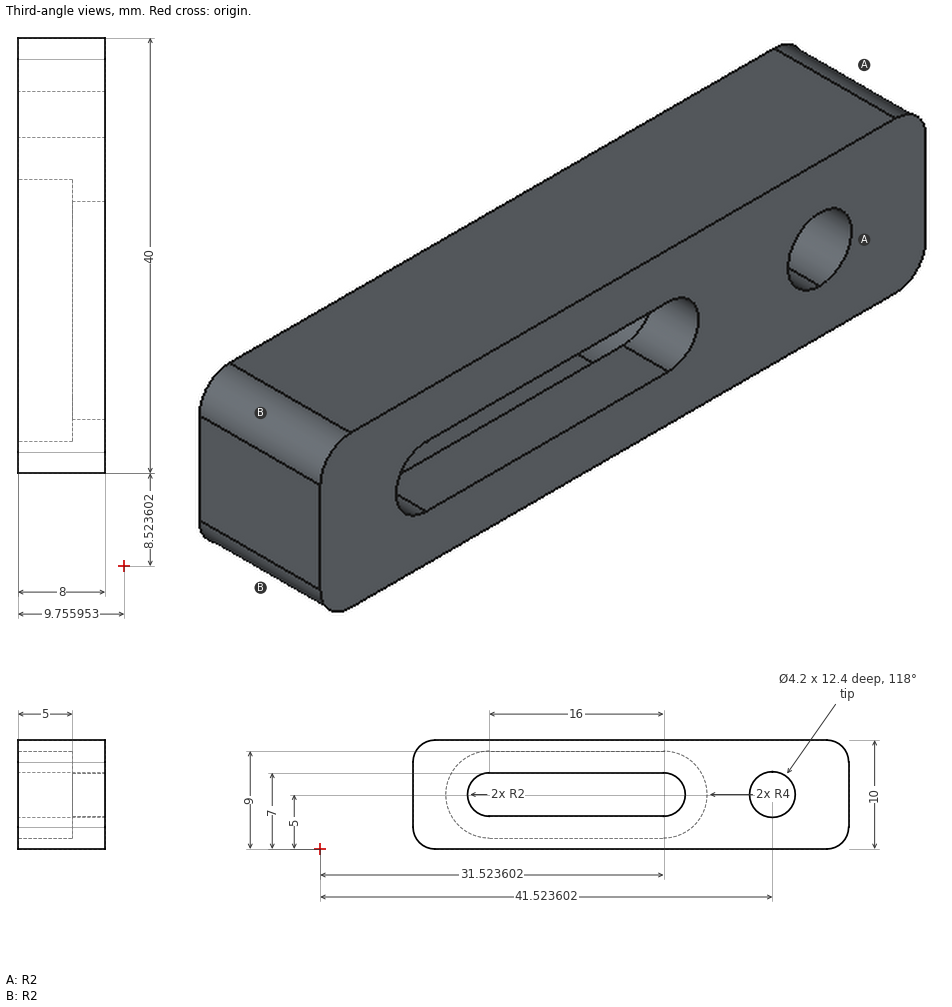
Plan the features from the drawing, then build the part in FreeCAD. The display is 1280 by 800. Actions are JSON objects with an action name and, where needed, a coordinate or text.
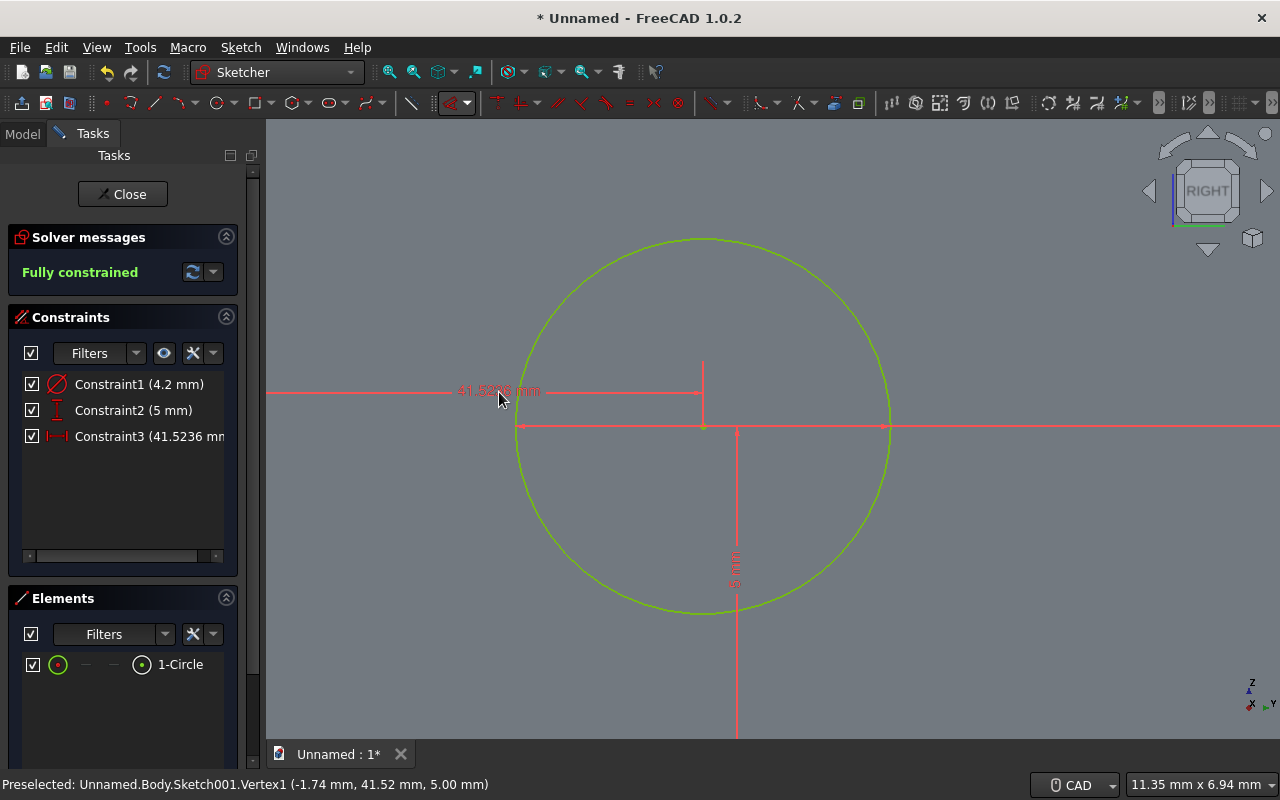
{"action": "left_click", "coordinate": [123, 194]}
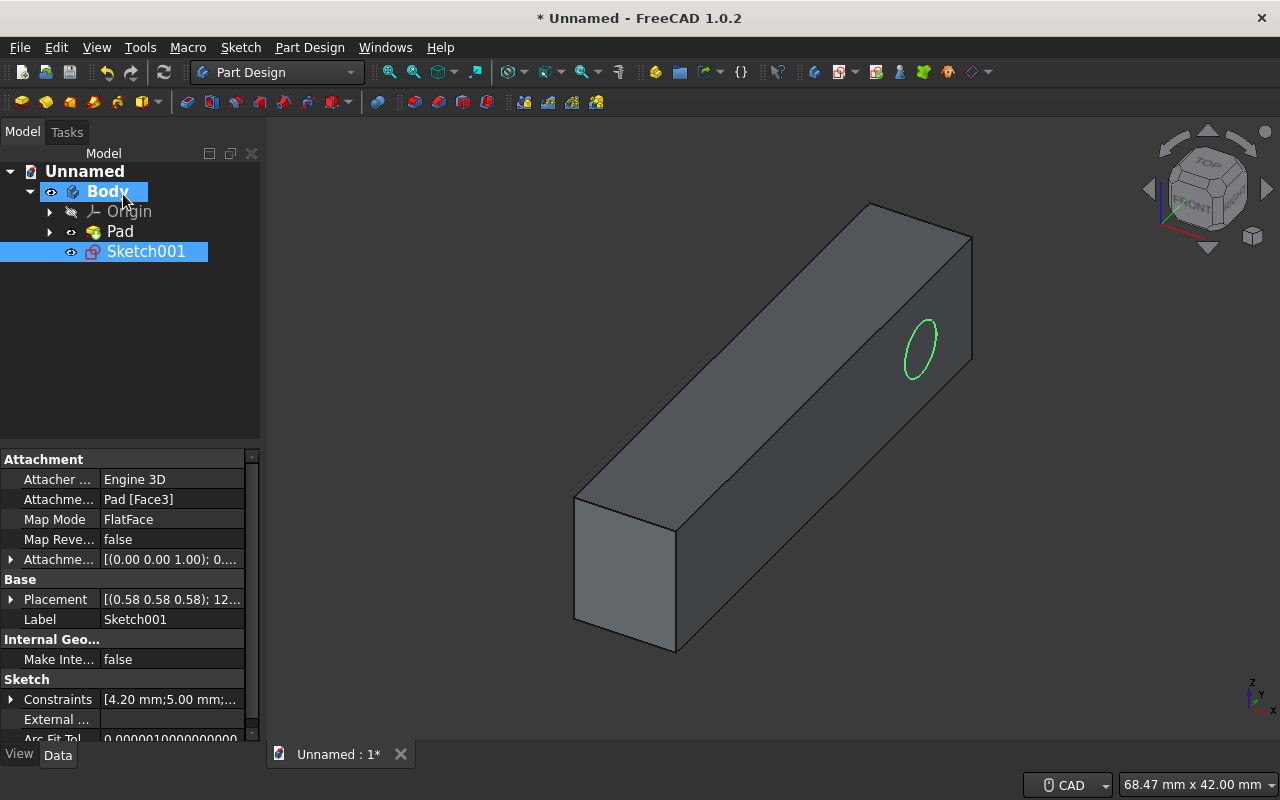
{"action": "left_click", "coordinate": [212, 102]}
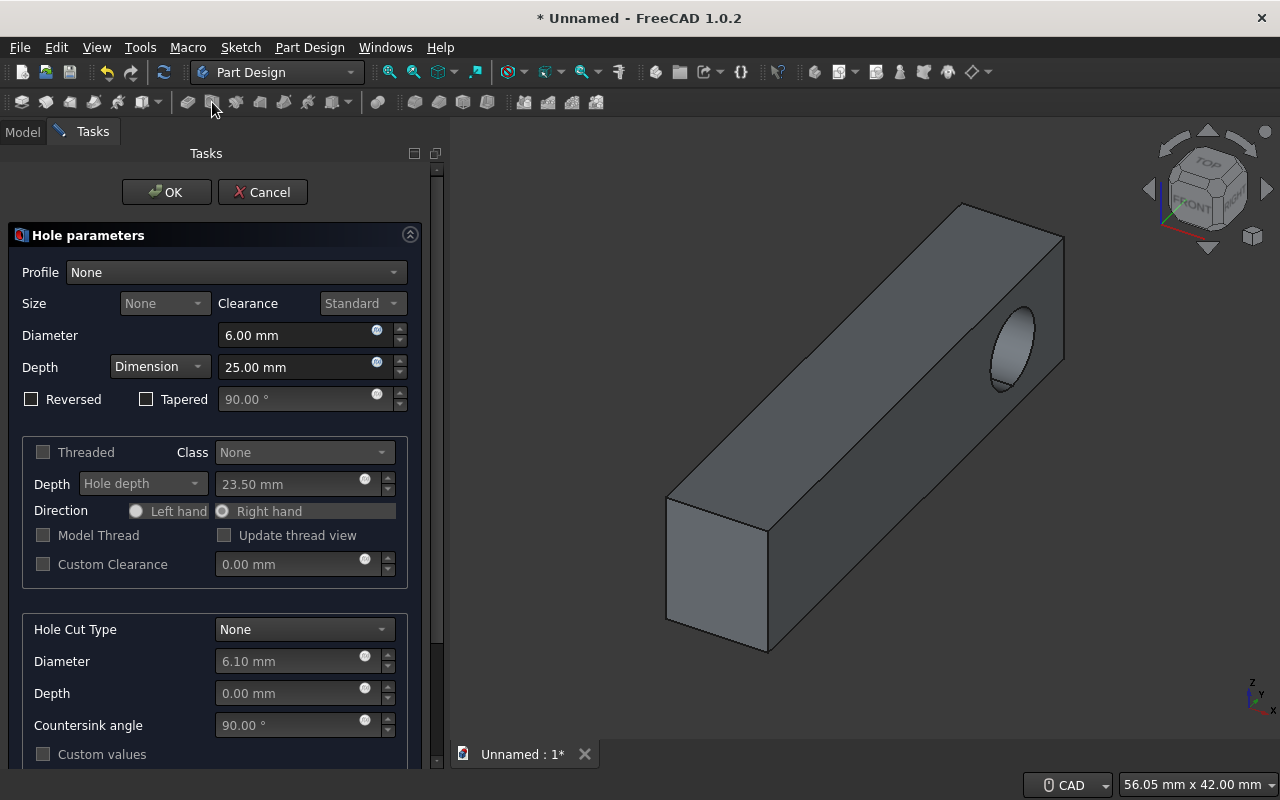
{"action": "triple_click", "coordinate": [305, 335]}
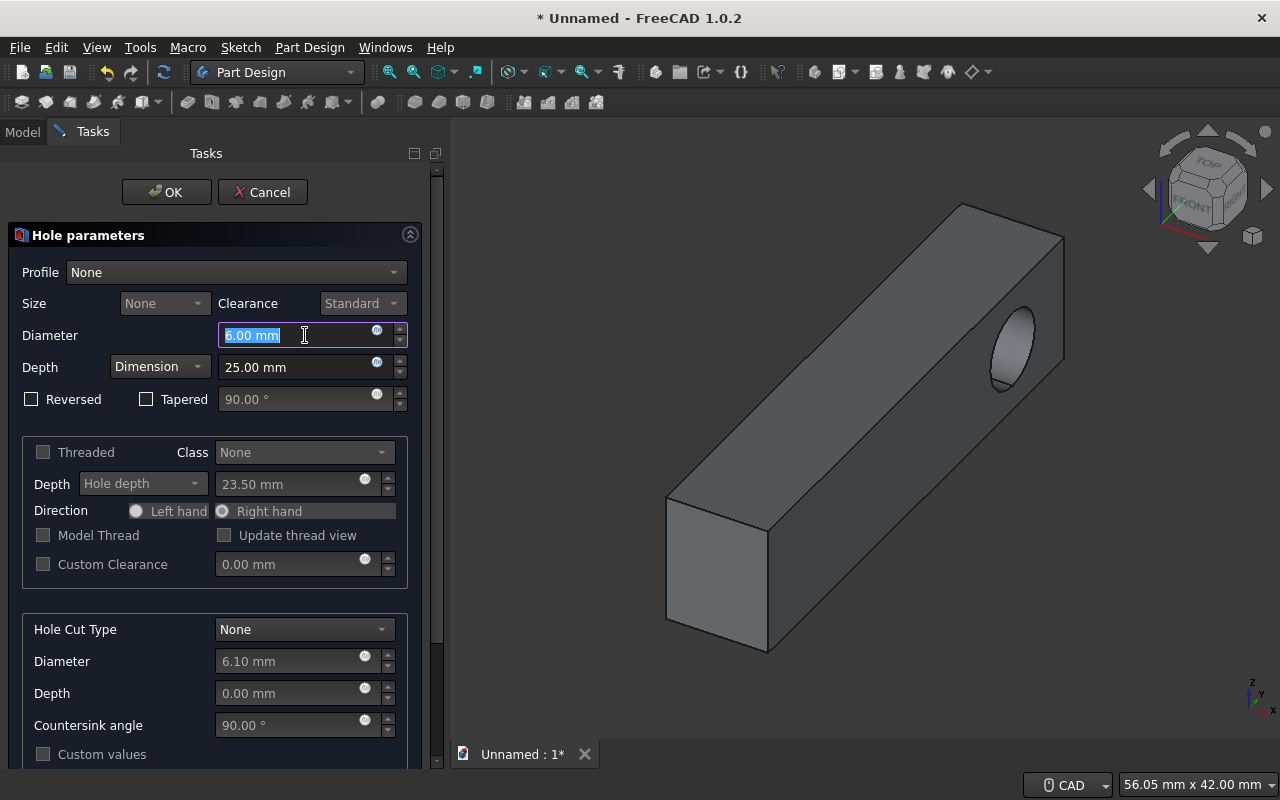
{"action": "type", "text": "4.2"}
{"action": "key", "text": "Tab"}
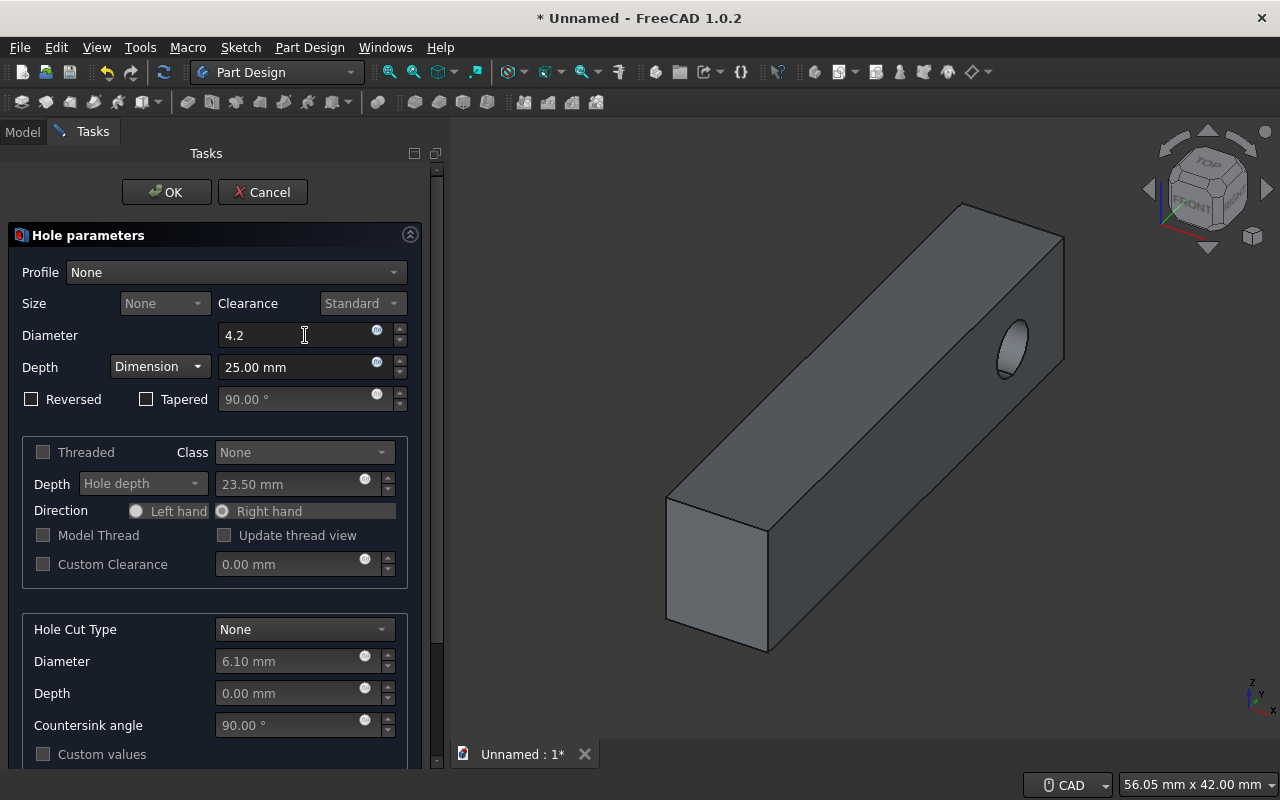
{"action": "triple_click", "coordinate": [305, 367]}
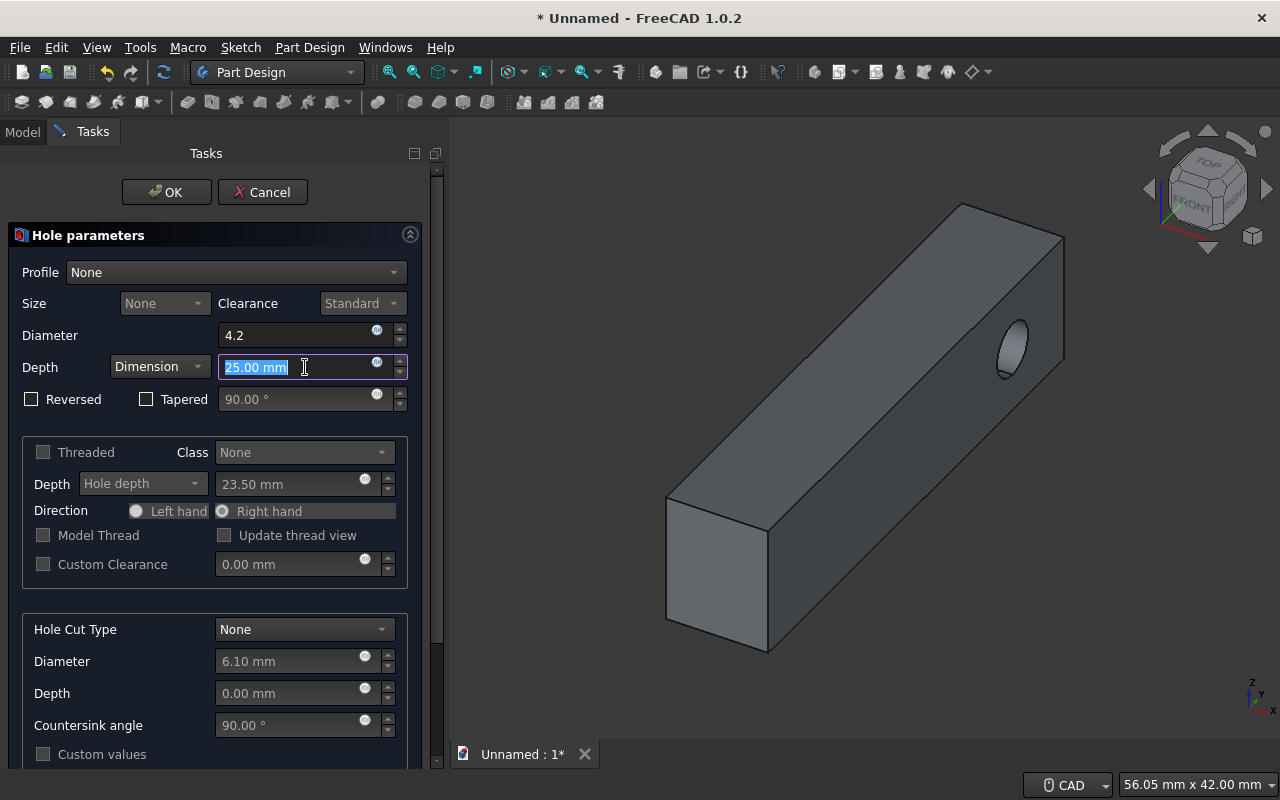
{"action": "type", "text": "12.4"}
{"action": "key", "text": "Tab"}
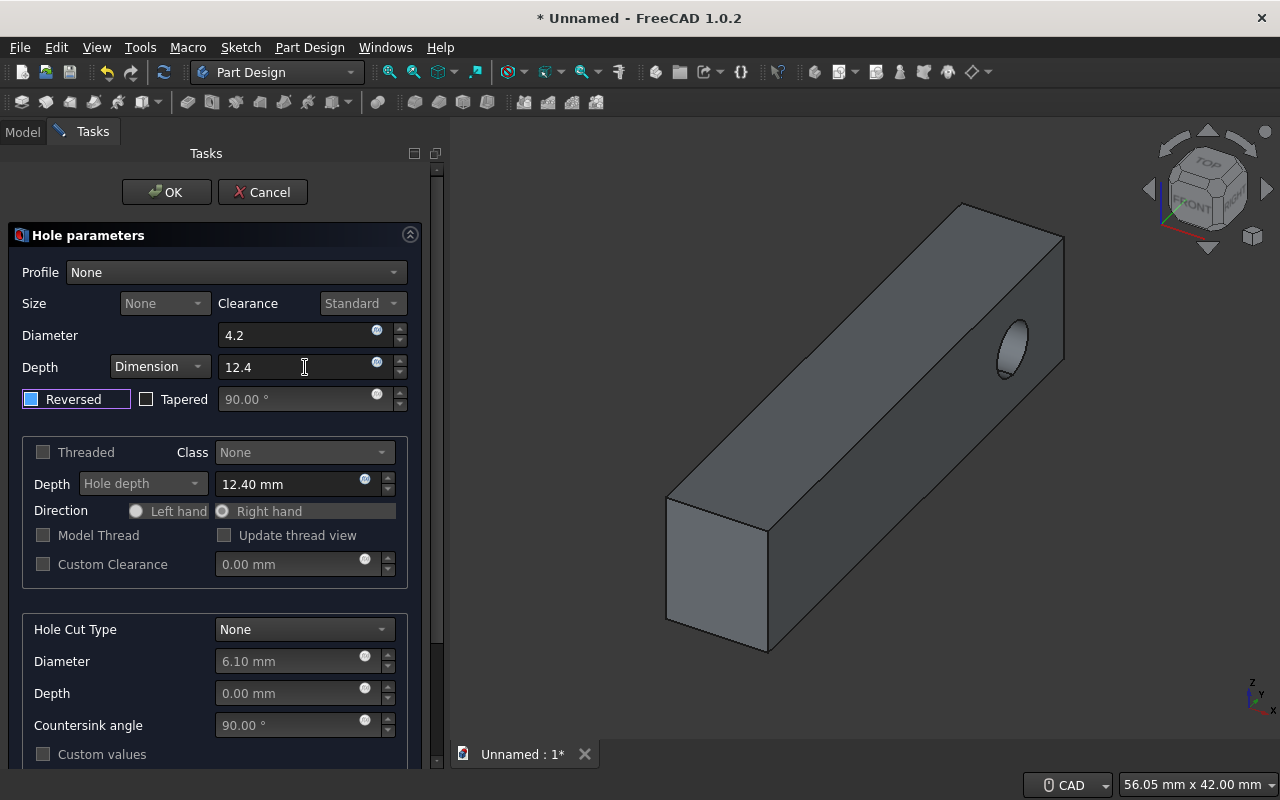
{"action": "left_click", "coordinate": [167, 192]}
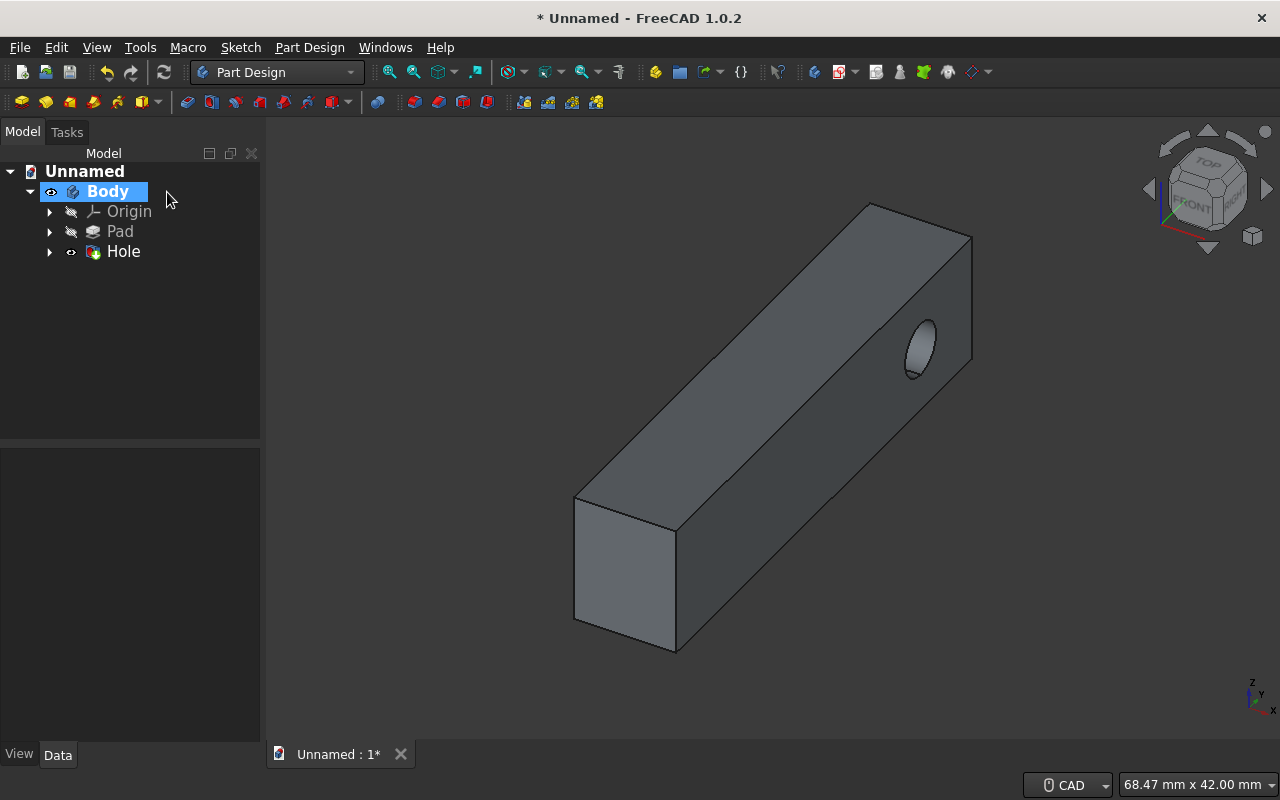
{"action": "key", "text": "0"}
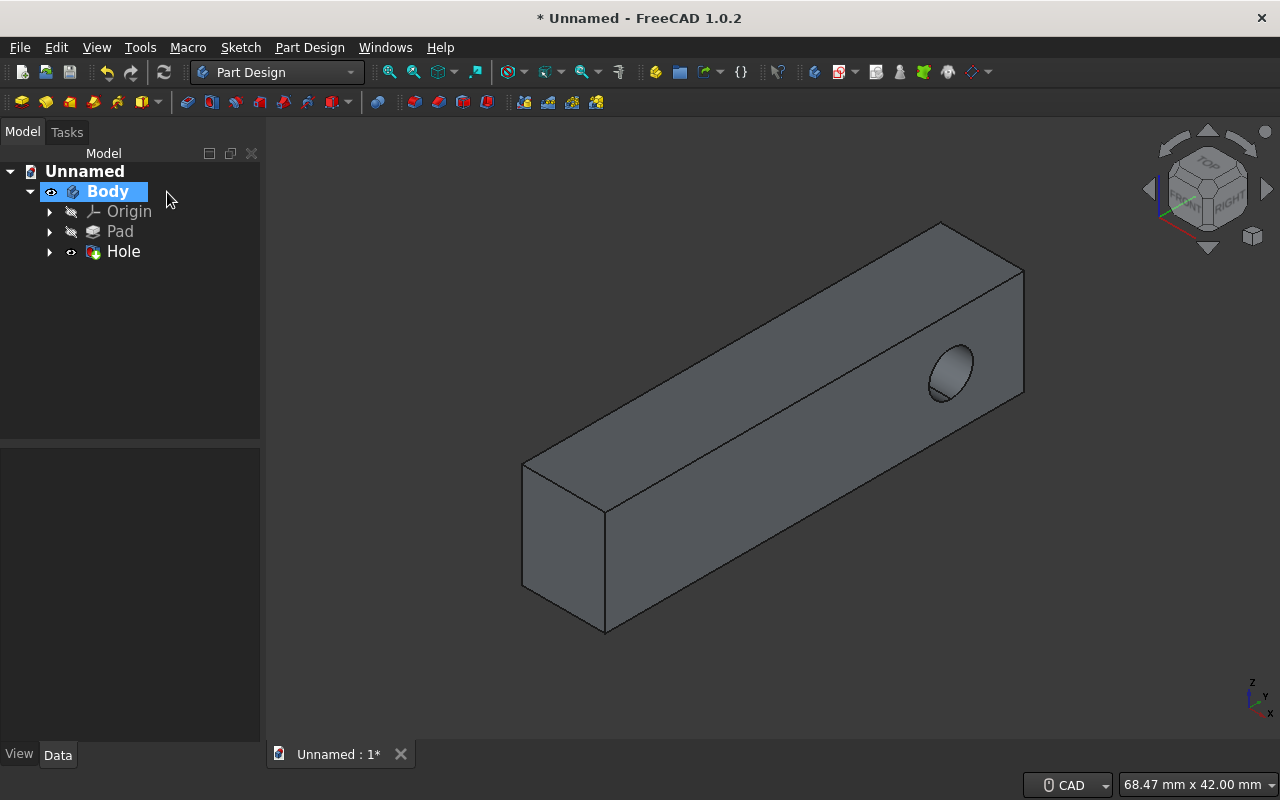
{"action": "key", "text": "2"}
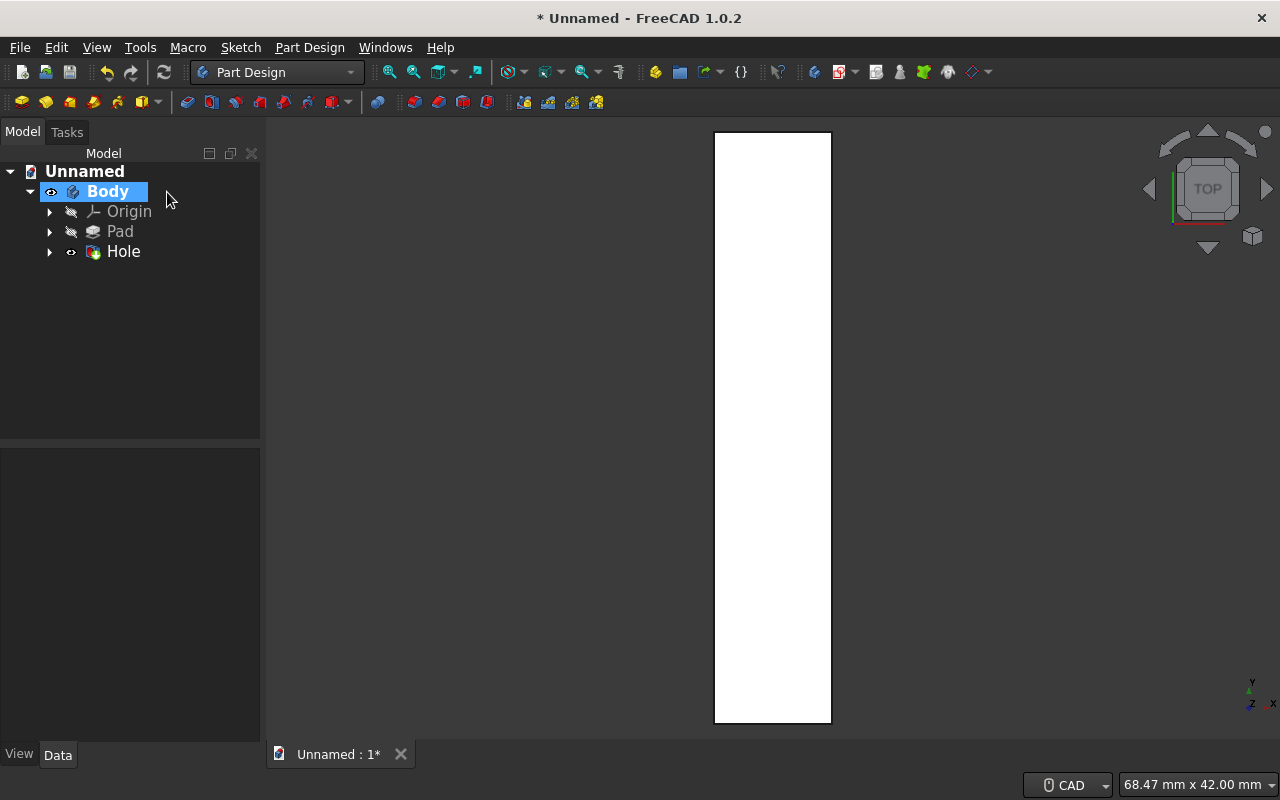
{"action": "key", "text": "1"}